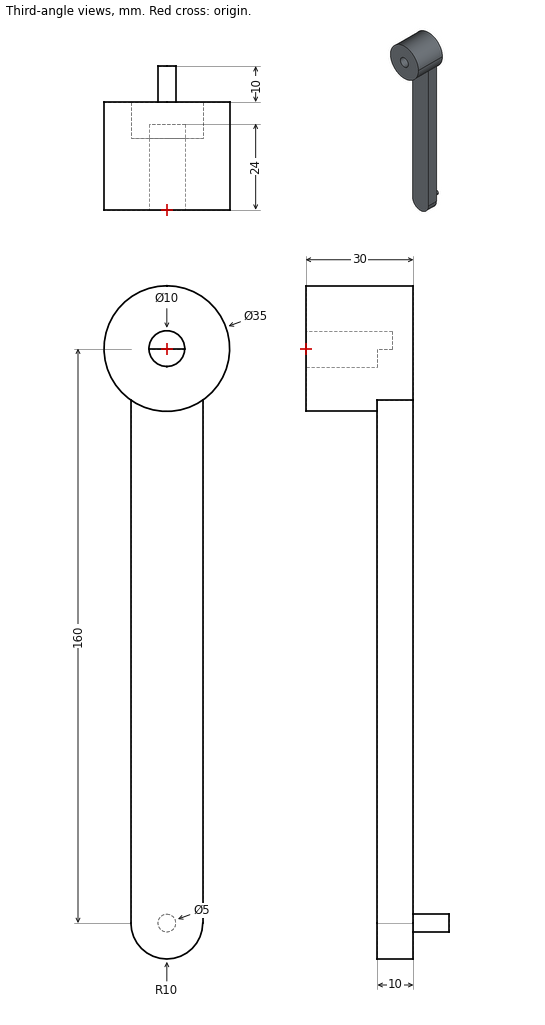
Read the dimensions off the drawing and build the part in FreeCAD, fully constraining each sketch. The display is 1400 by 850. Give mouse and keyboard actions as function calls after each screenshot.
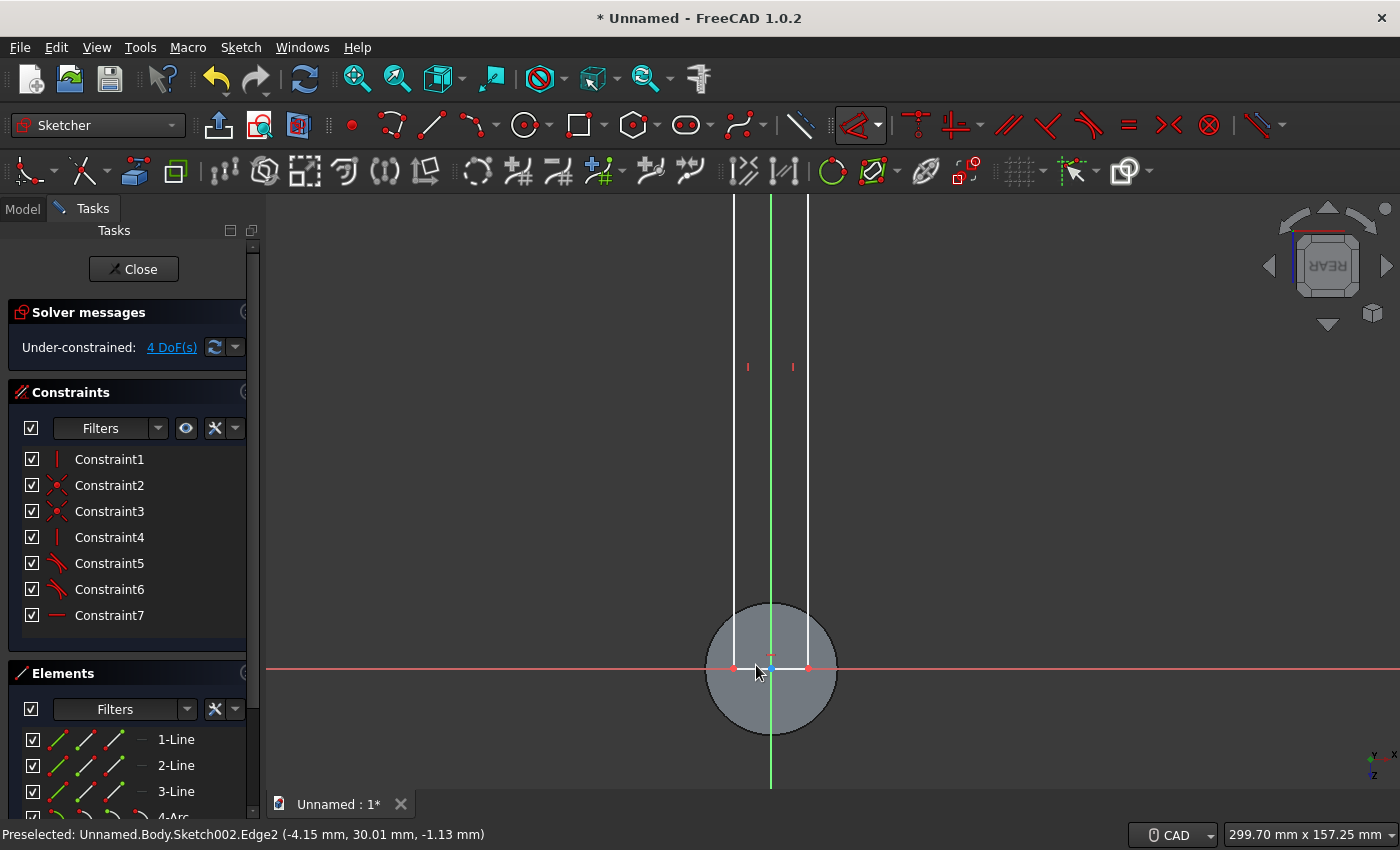
scroll(756, 667, down, 3)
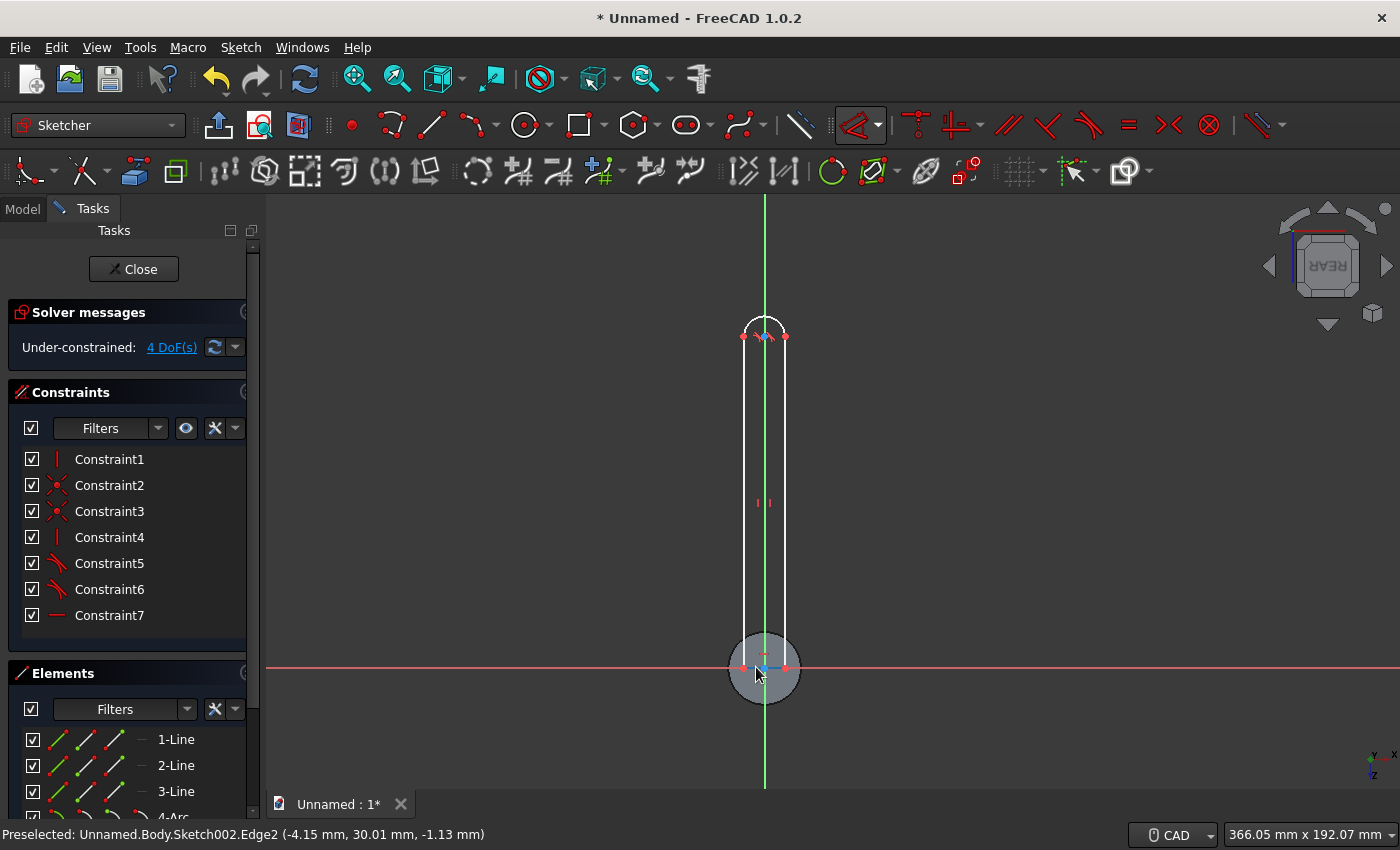
click(765, 337)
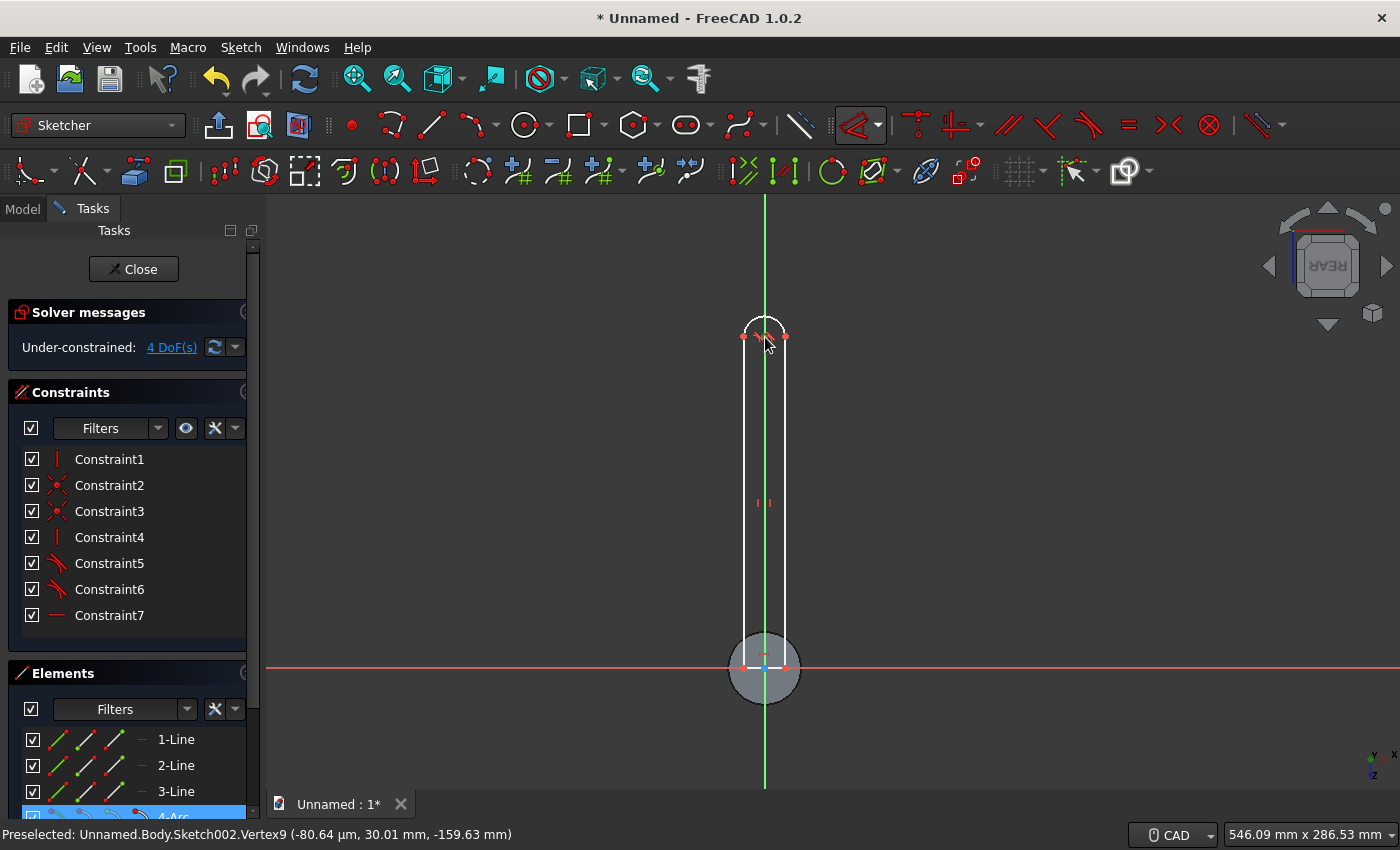
click(765, 722)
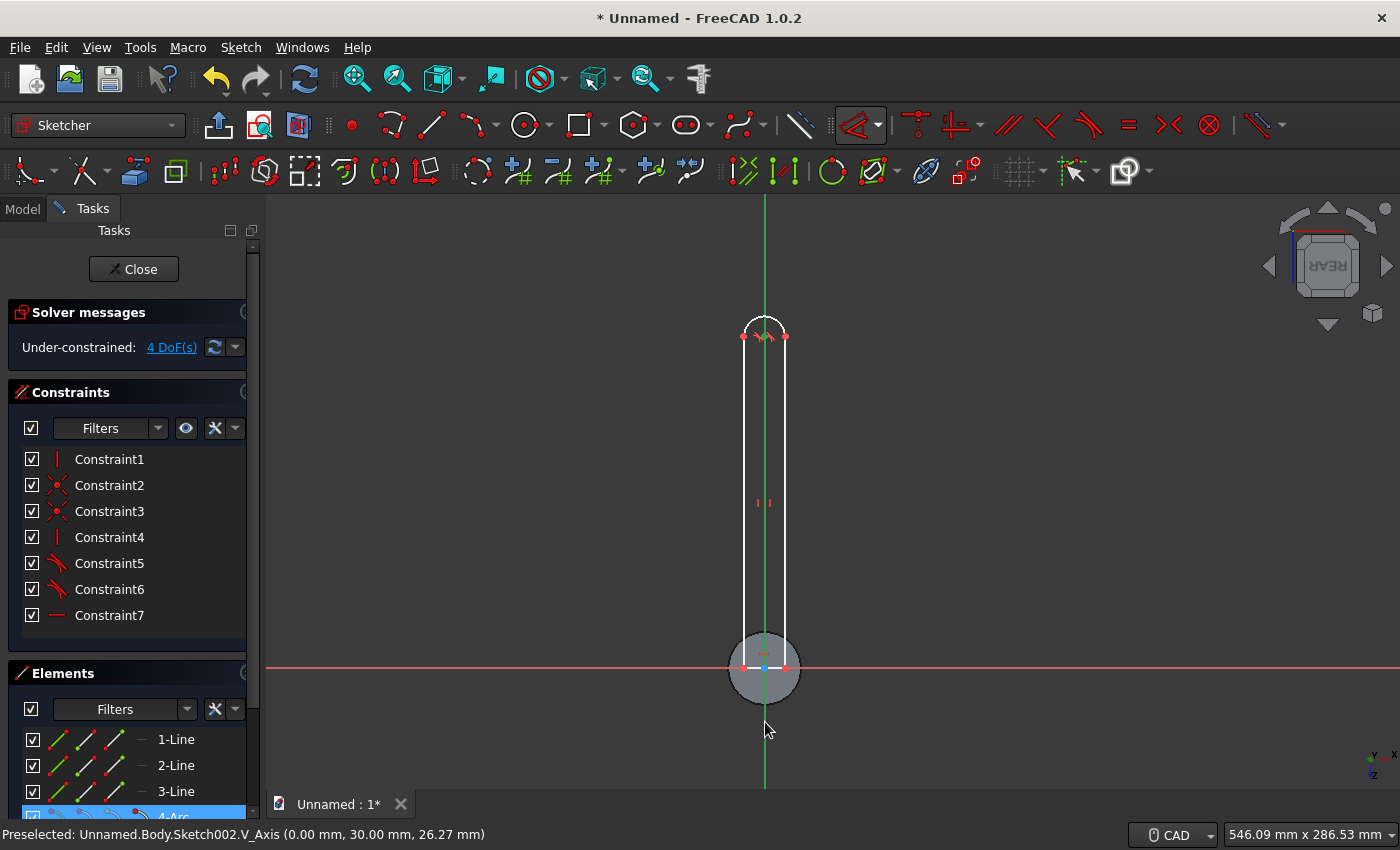
key(c)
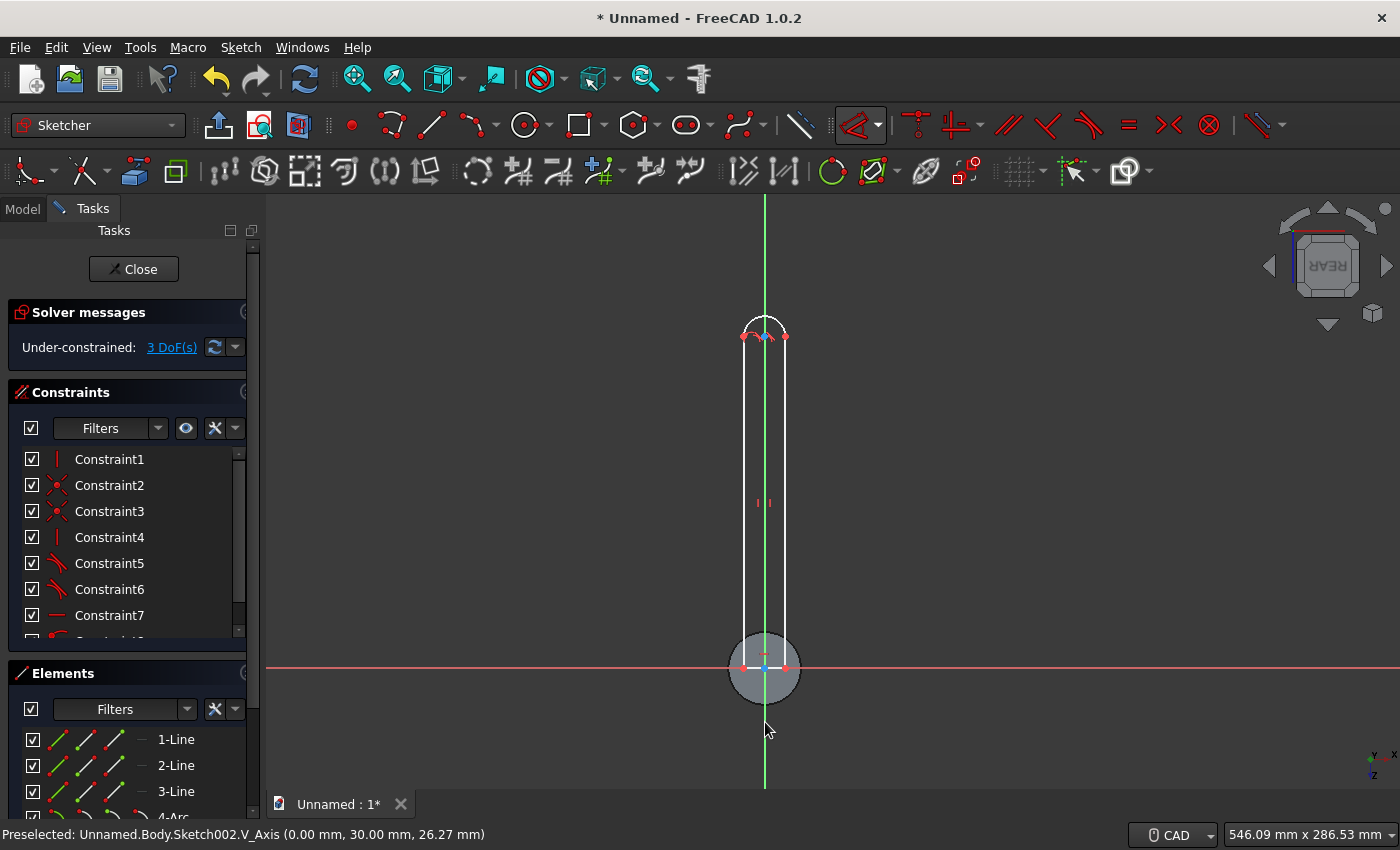
key(d)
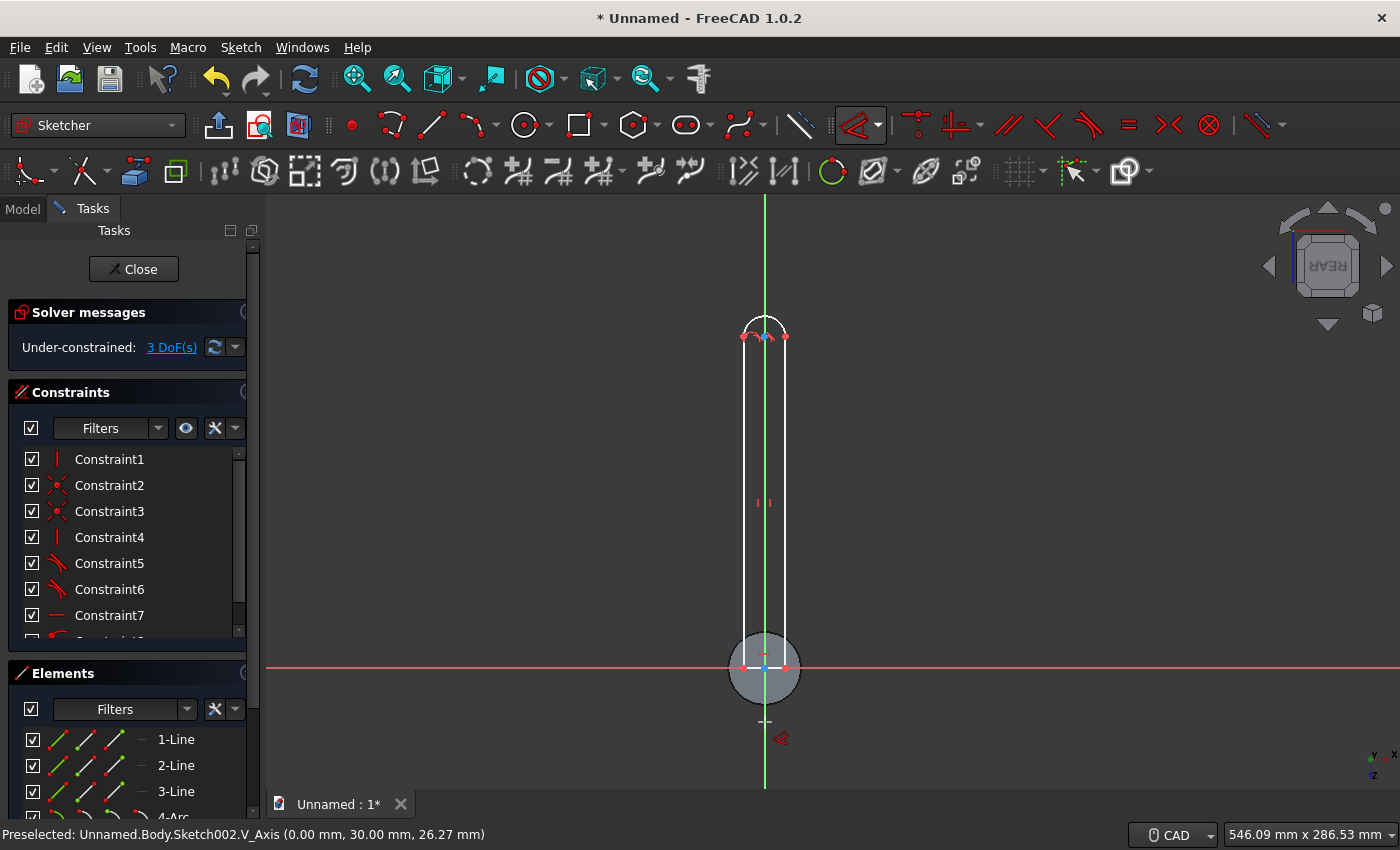
scroll(777, 320, up, 4)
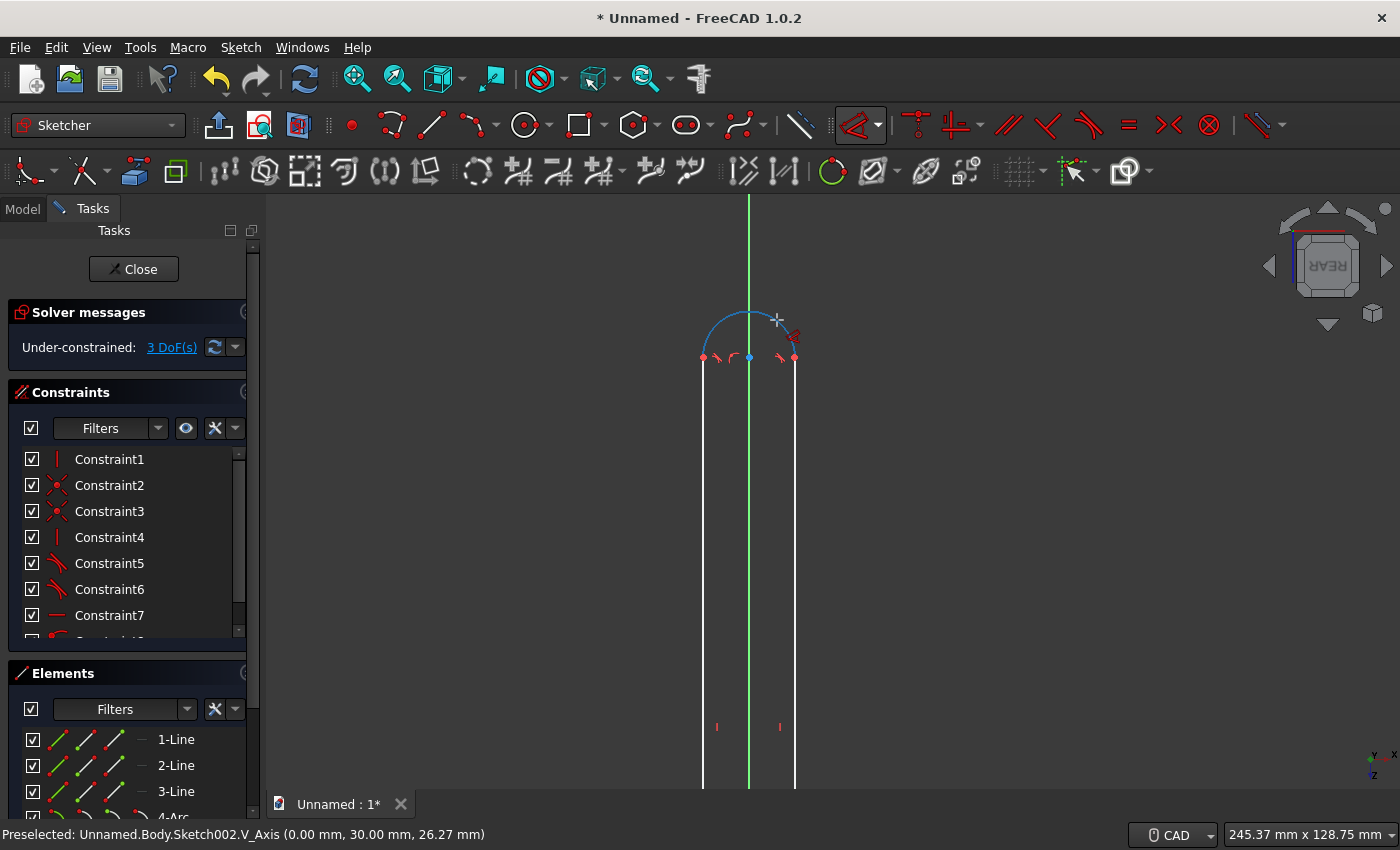
click(776, 320)
click(795, 294)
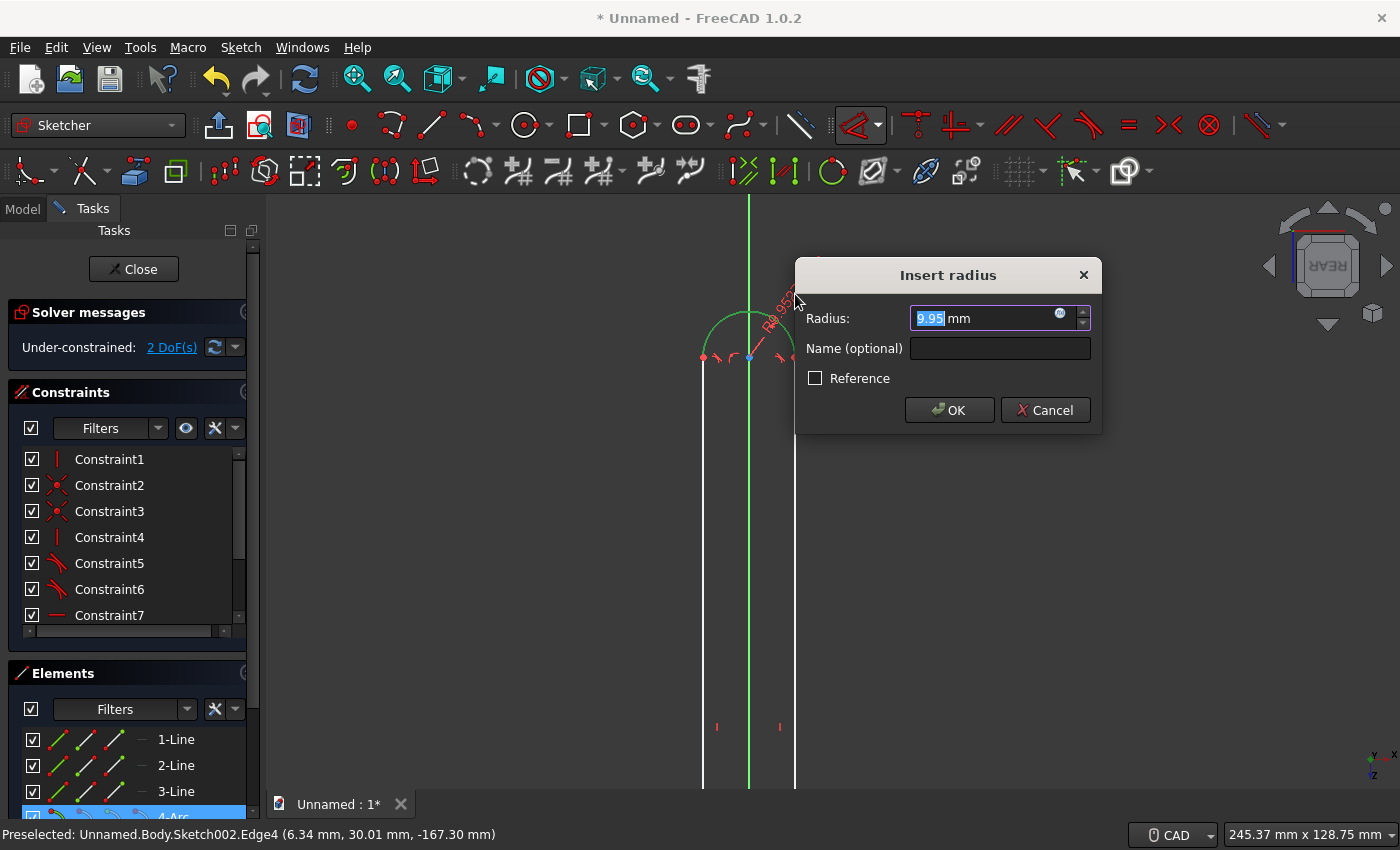
text(10)
key(Return)
key(Escape)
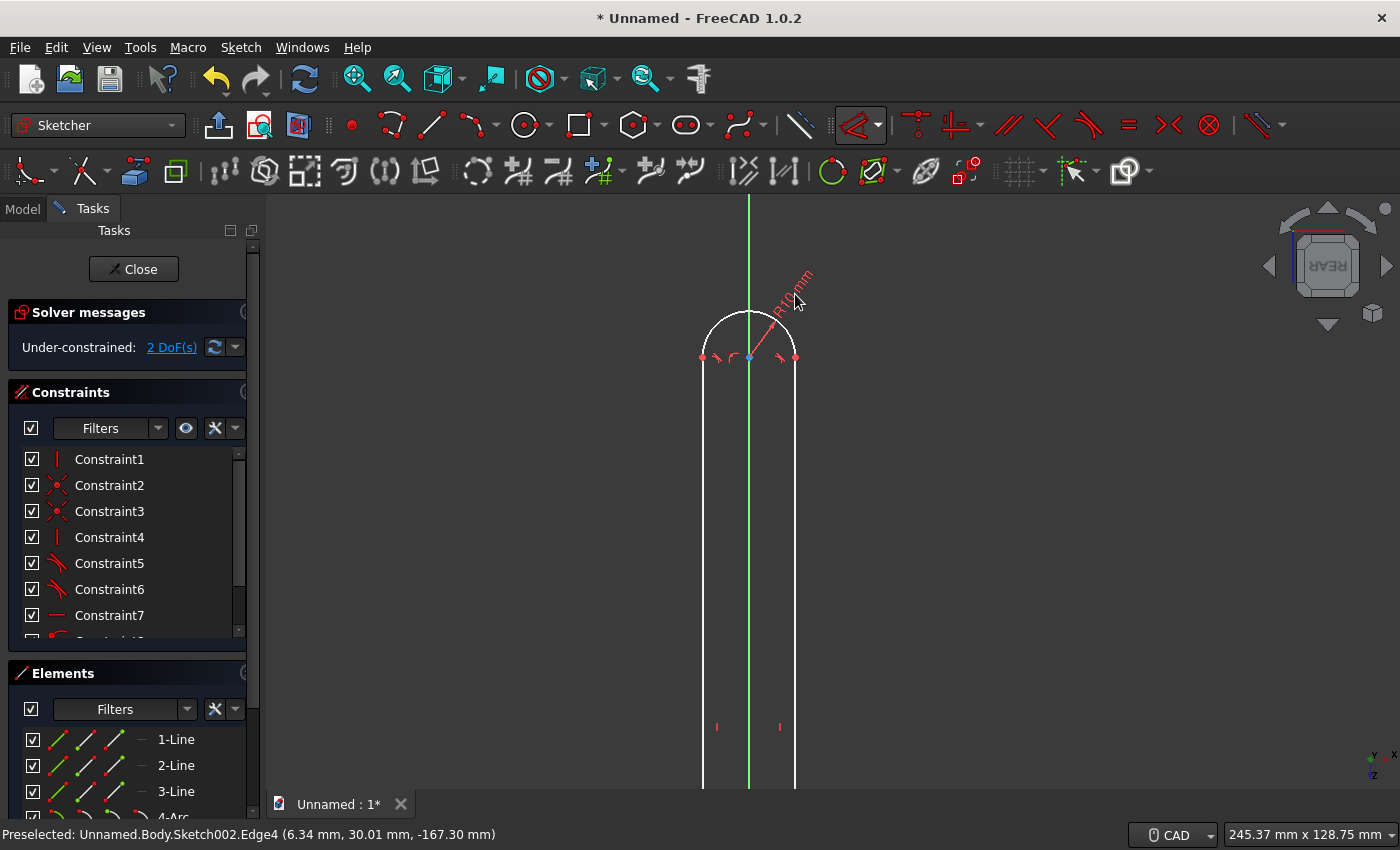
scroll(777, 319, down, 4)